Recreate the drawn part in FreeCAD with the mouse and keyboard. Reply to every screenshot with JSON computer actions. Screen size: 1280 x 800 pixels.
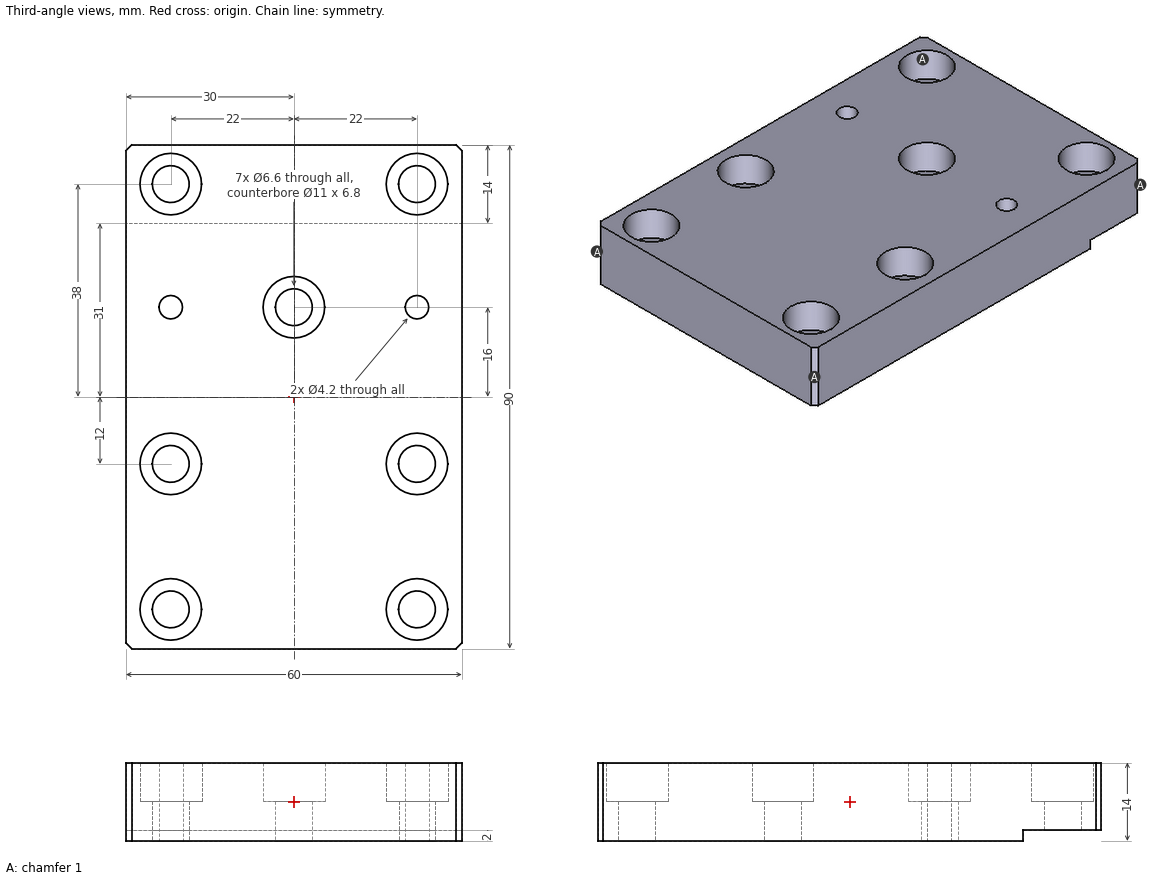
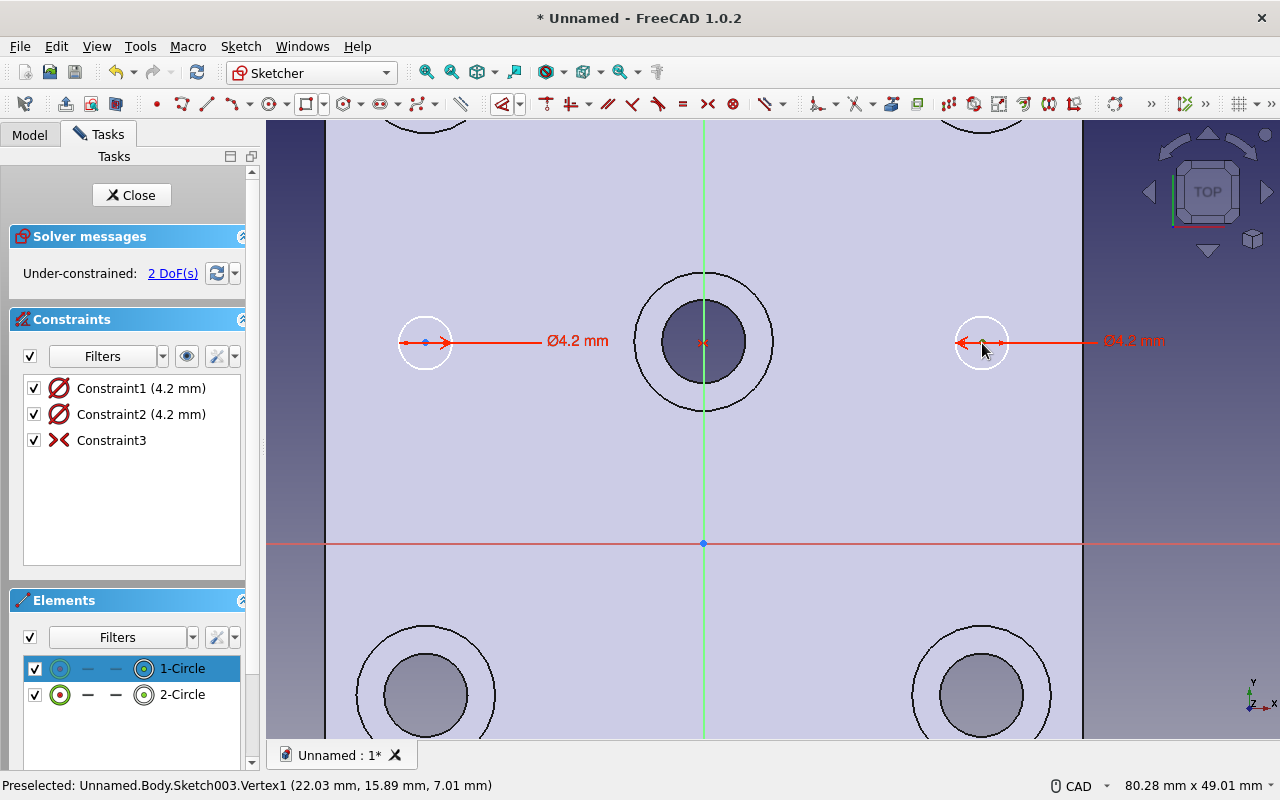
{"action": "left_click", "coordinate": [520, 104]}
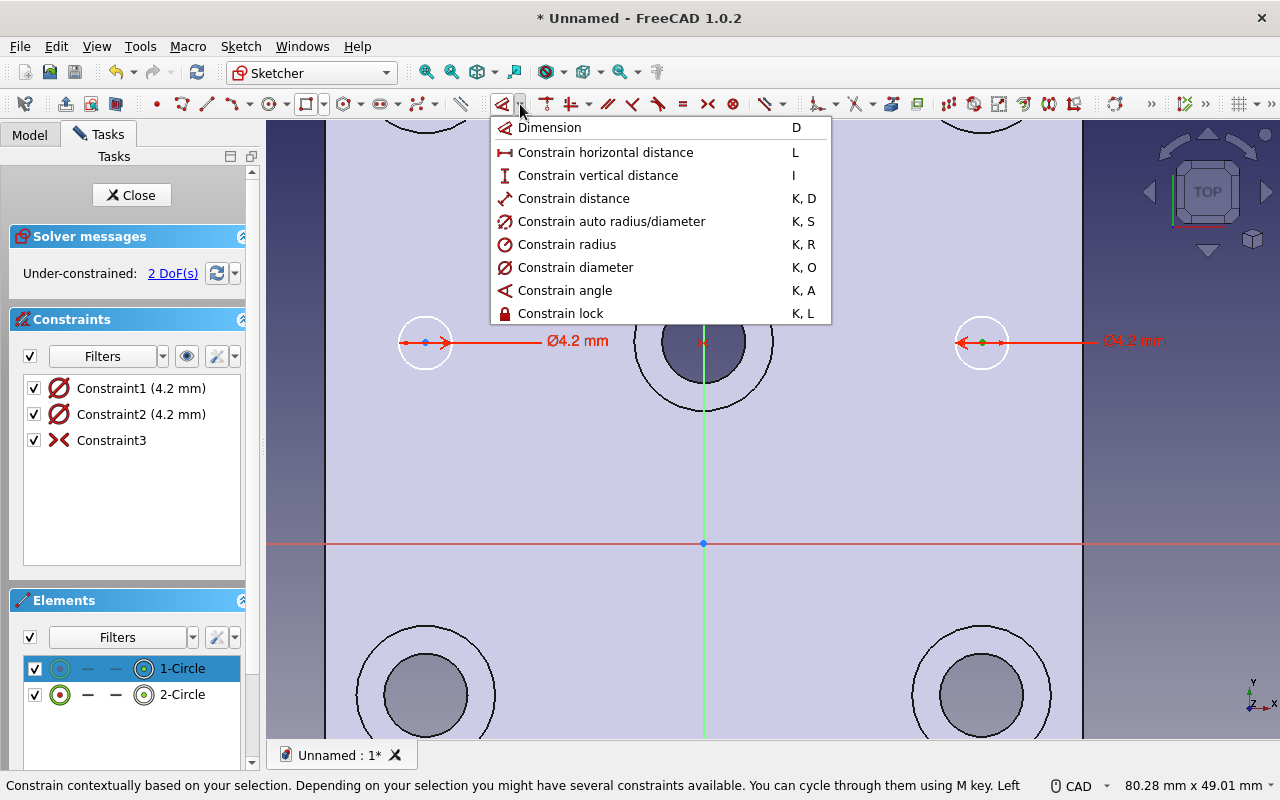
{"action": "left_click", "coordinate": [661, 152]}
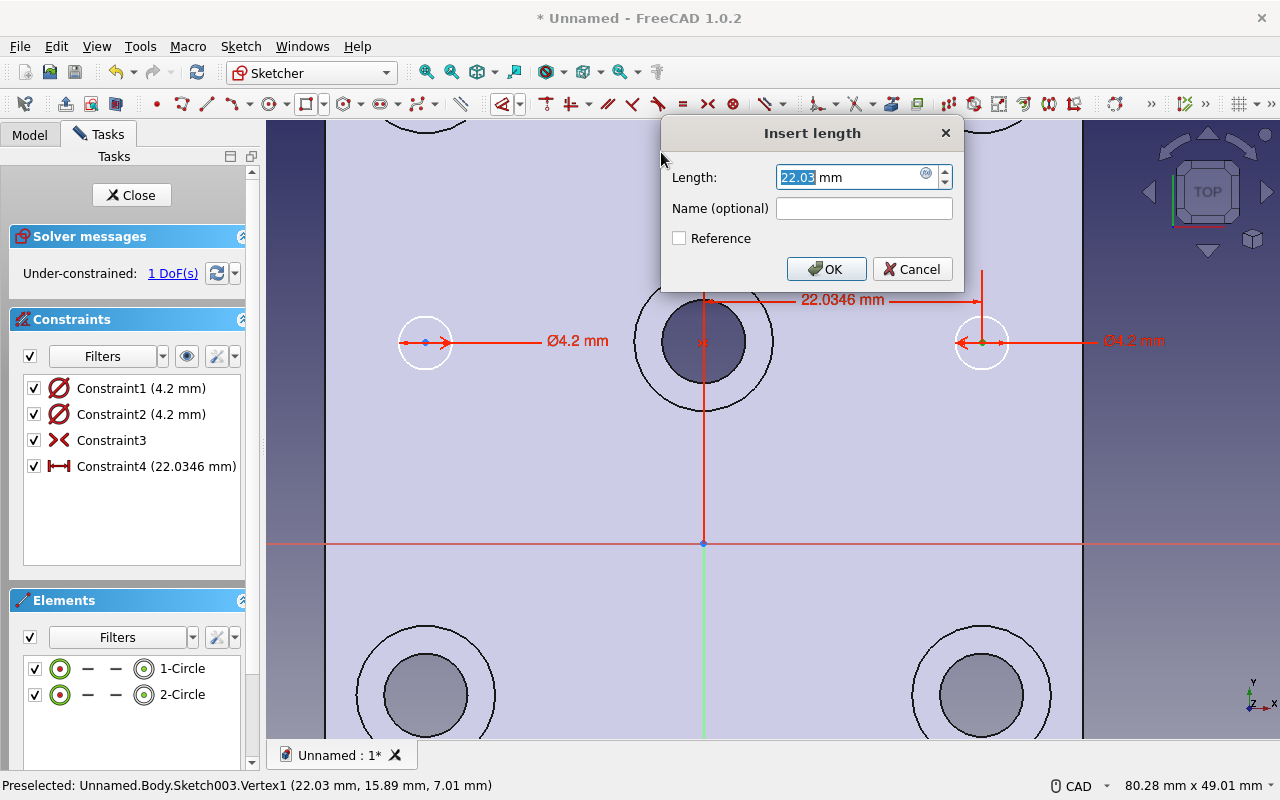
{"action": "type", "text": "22"}
{"action": "key", "text": "Return"}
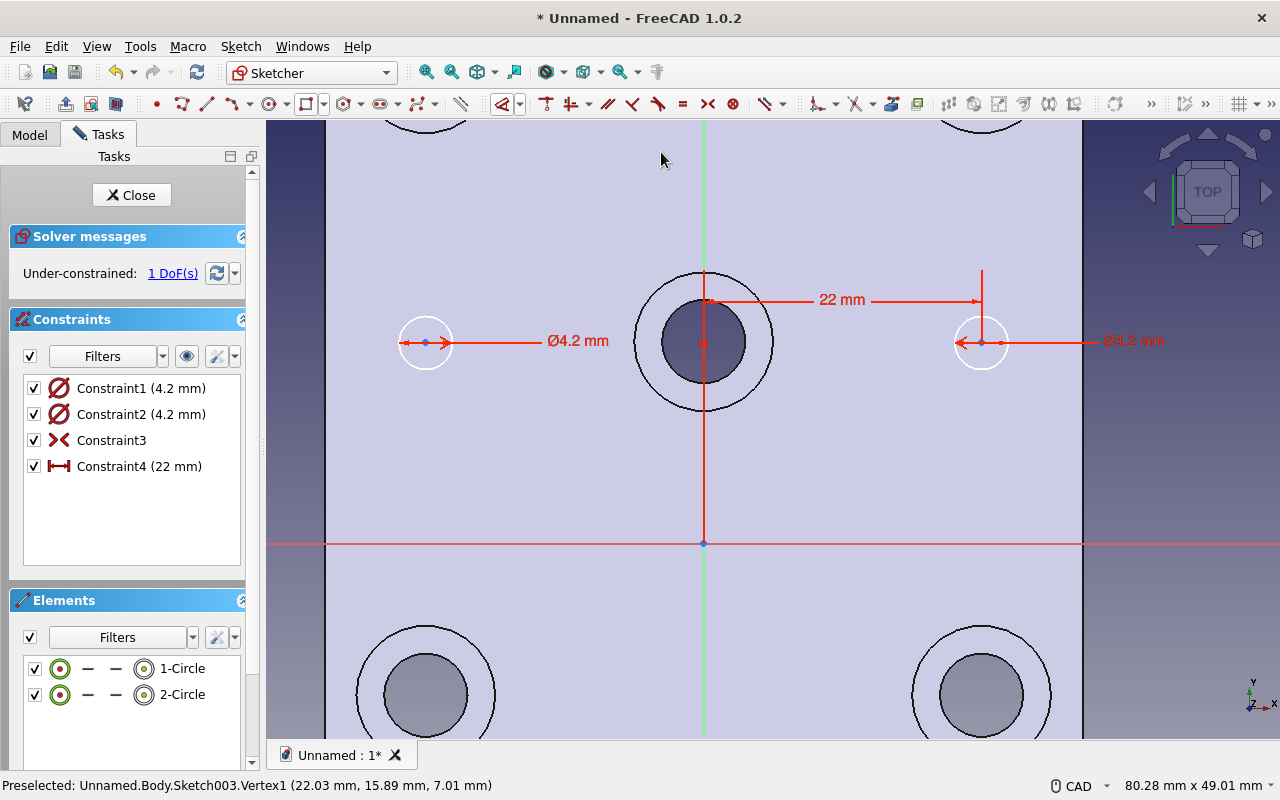
{"action": "left_click", "coordinate": [982, 343]}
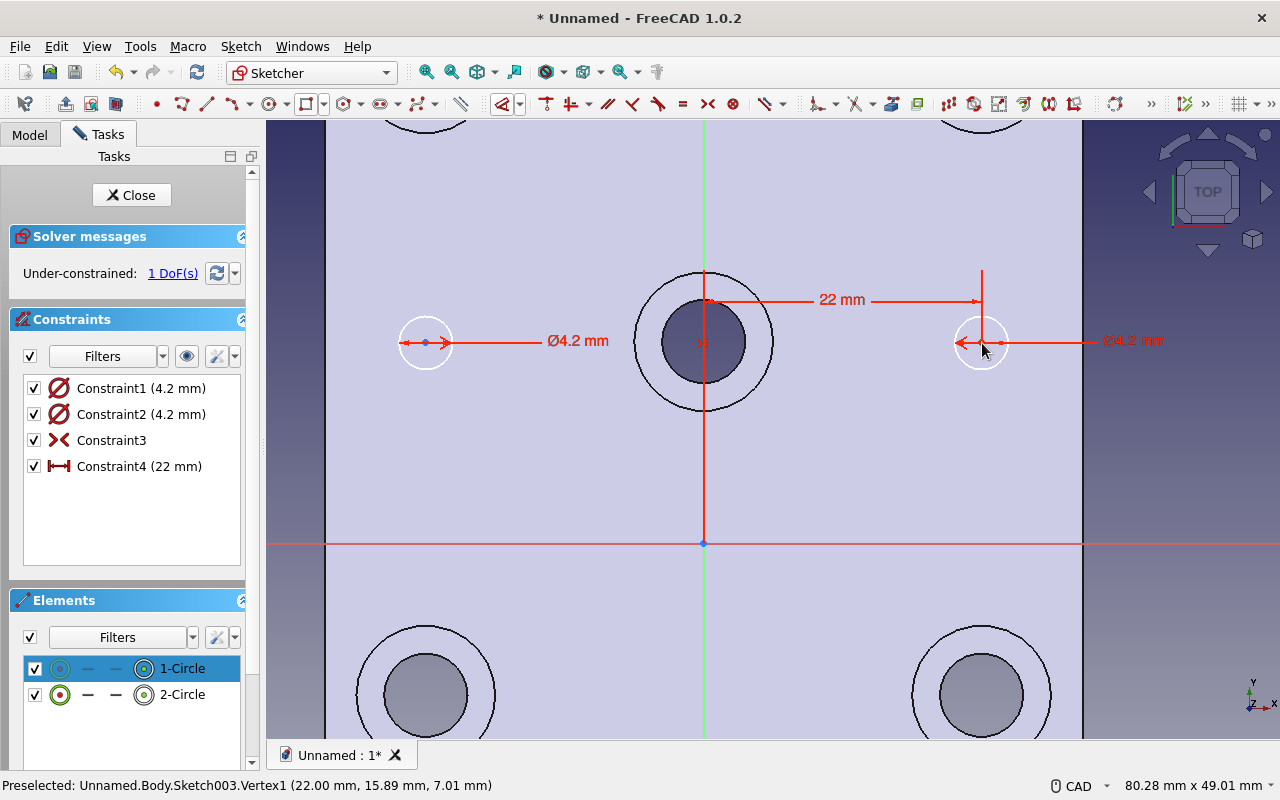
{"action": "left_click", "coordinate": [520, 104]}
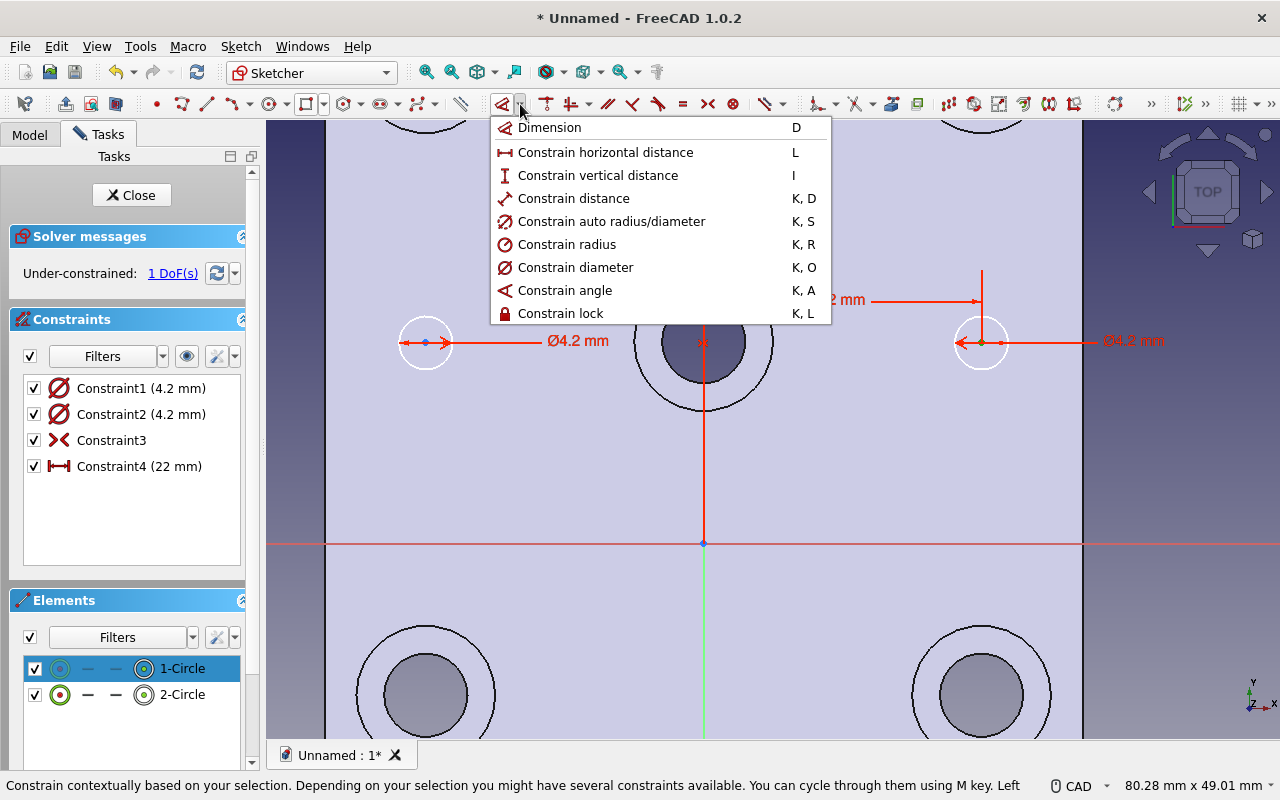
{"action": "left_click", "coordinate": [661, 176]}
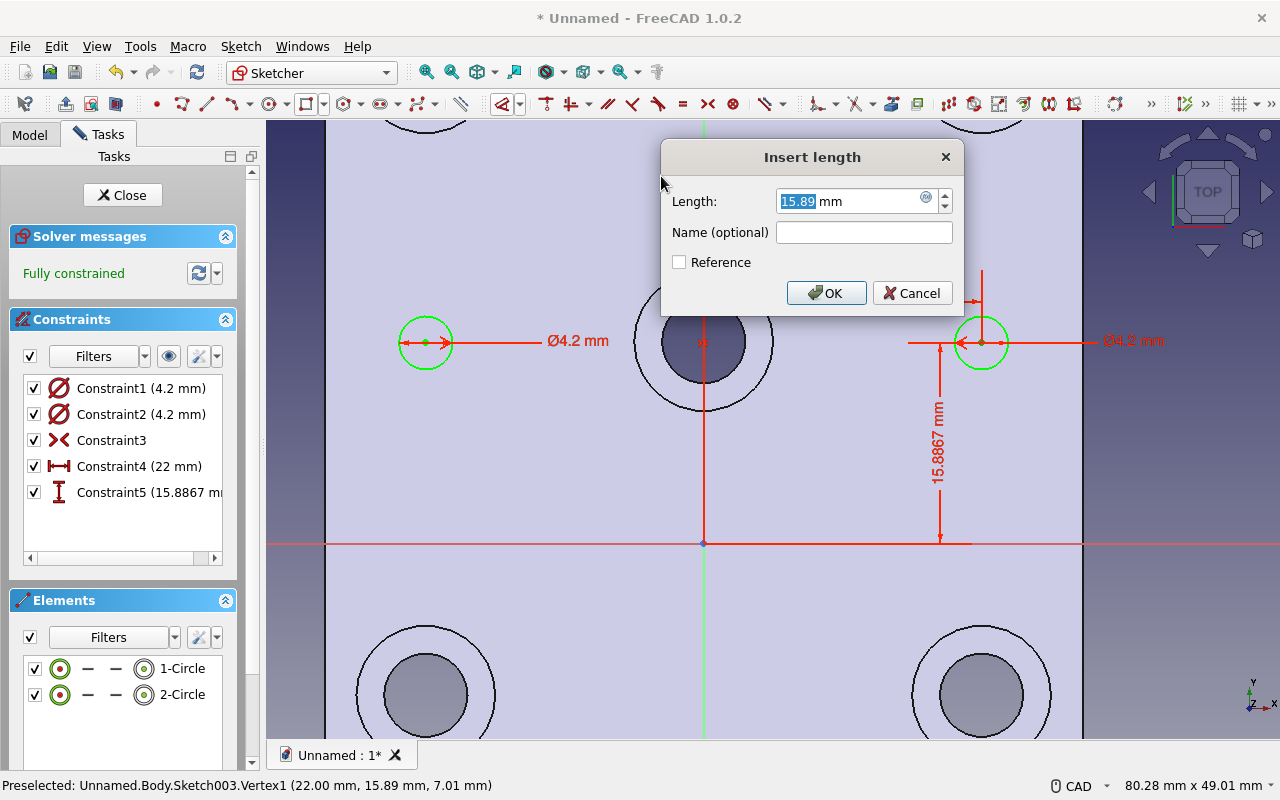
{"action": "type", "text": "16"}
{"action": "key", "text": "Return"}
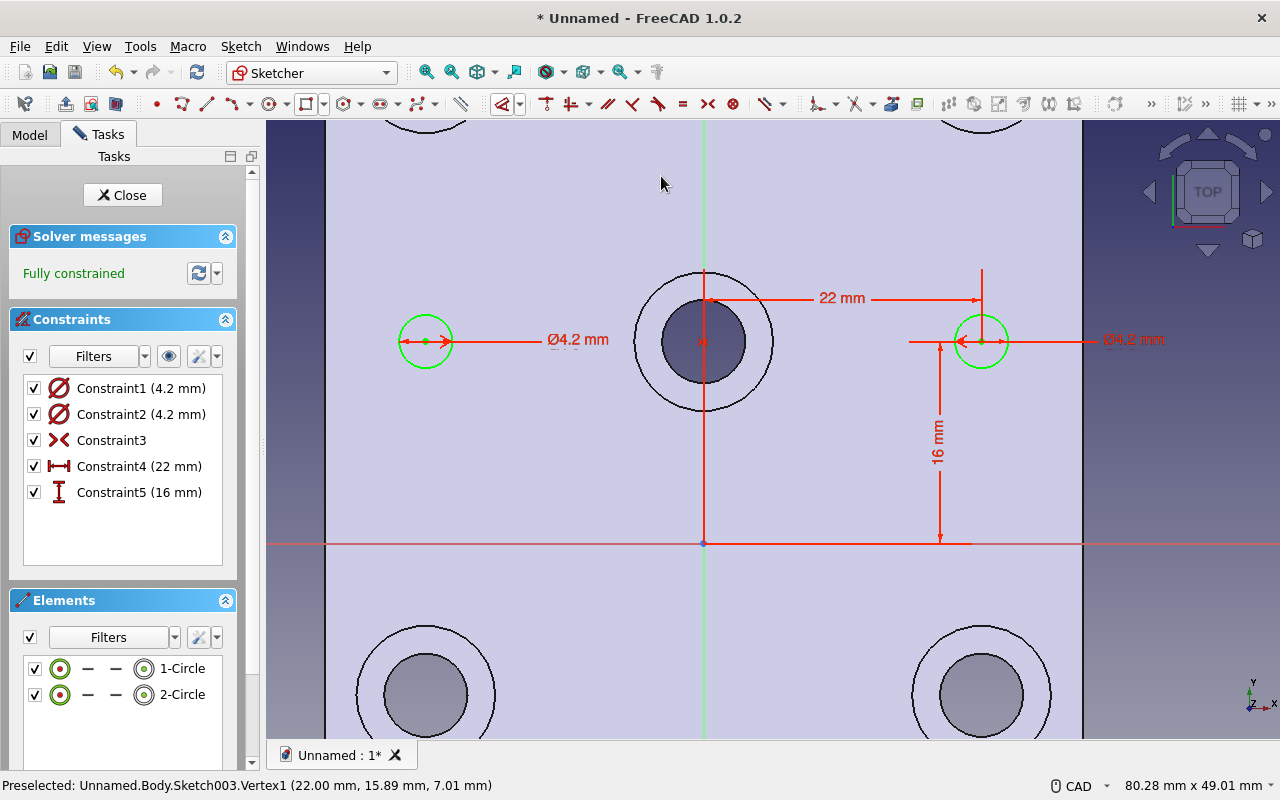
{"action": "left_click", "coordinate": [123, 195]}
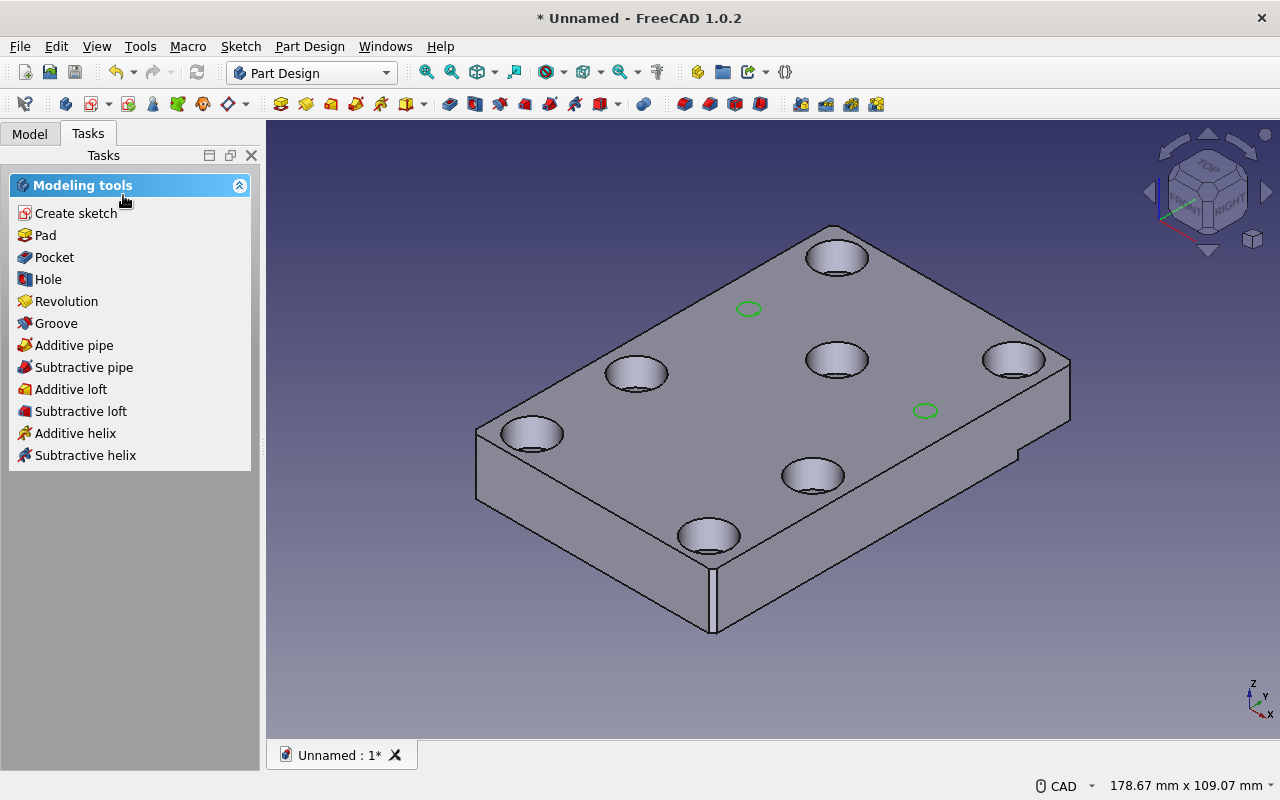
{"action": "left_click", "coordinate": [475, 104]}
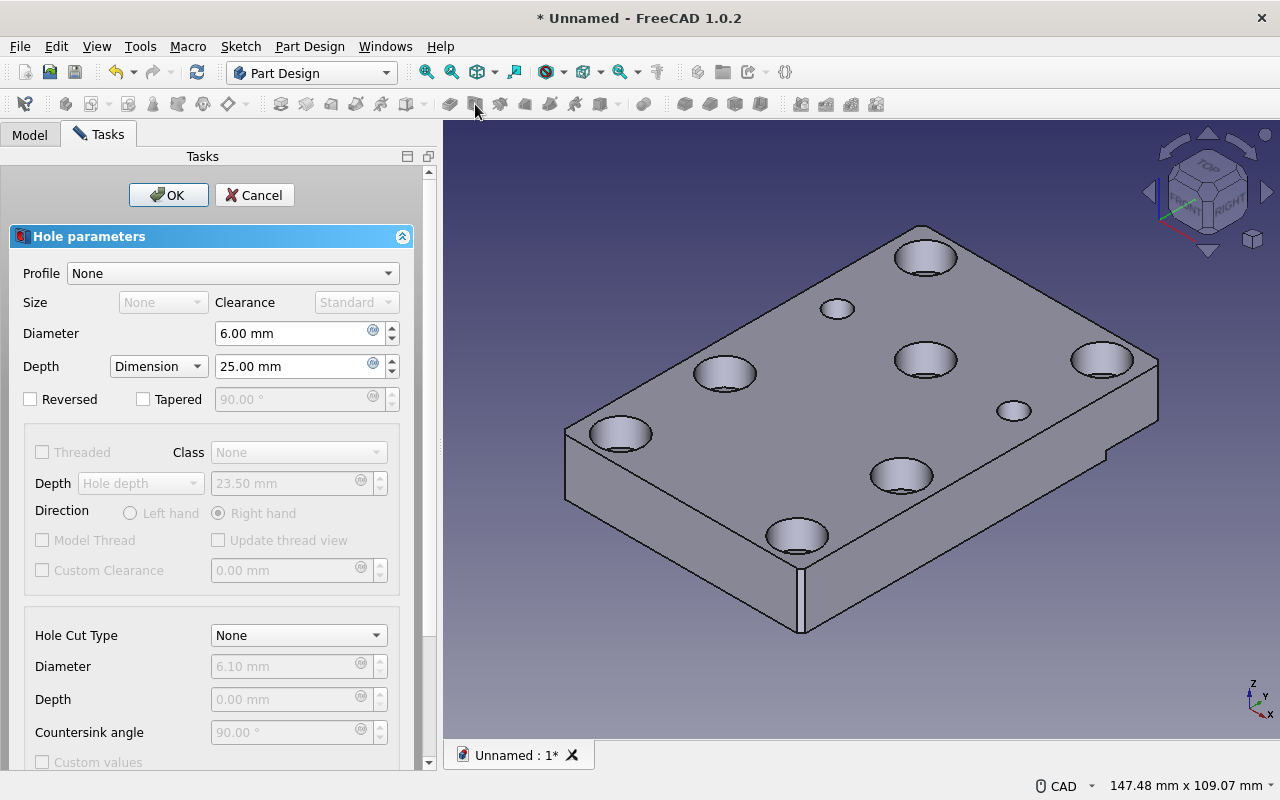
{"action": "triple_click", "coordinate": [300, 334]}